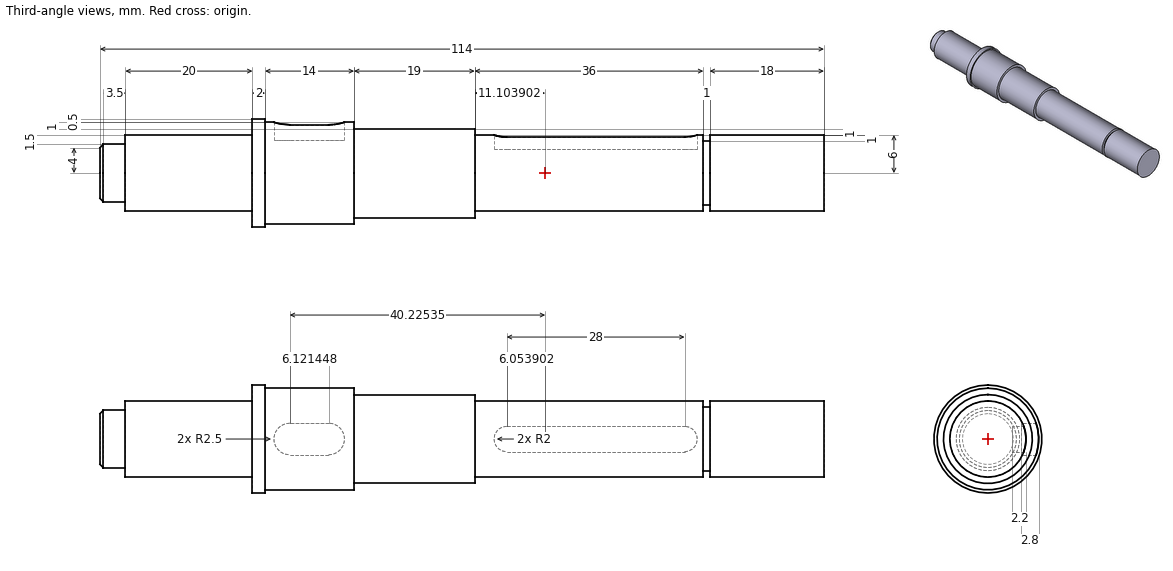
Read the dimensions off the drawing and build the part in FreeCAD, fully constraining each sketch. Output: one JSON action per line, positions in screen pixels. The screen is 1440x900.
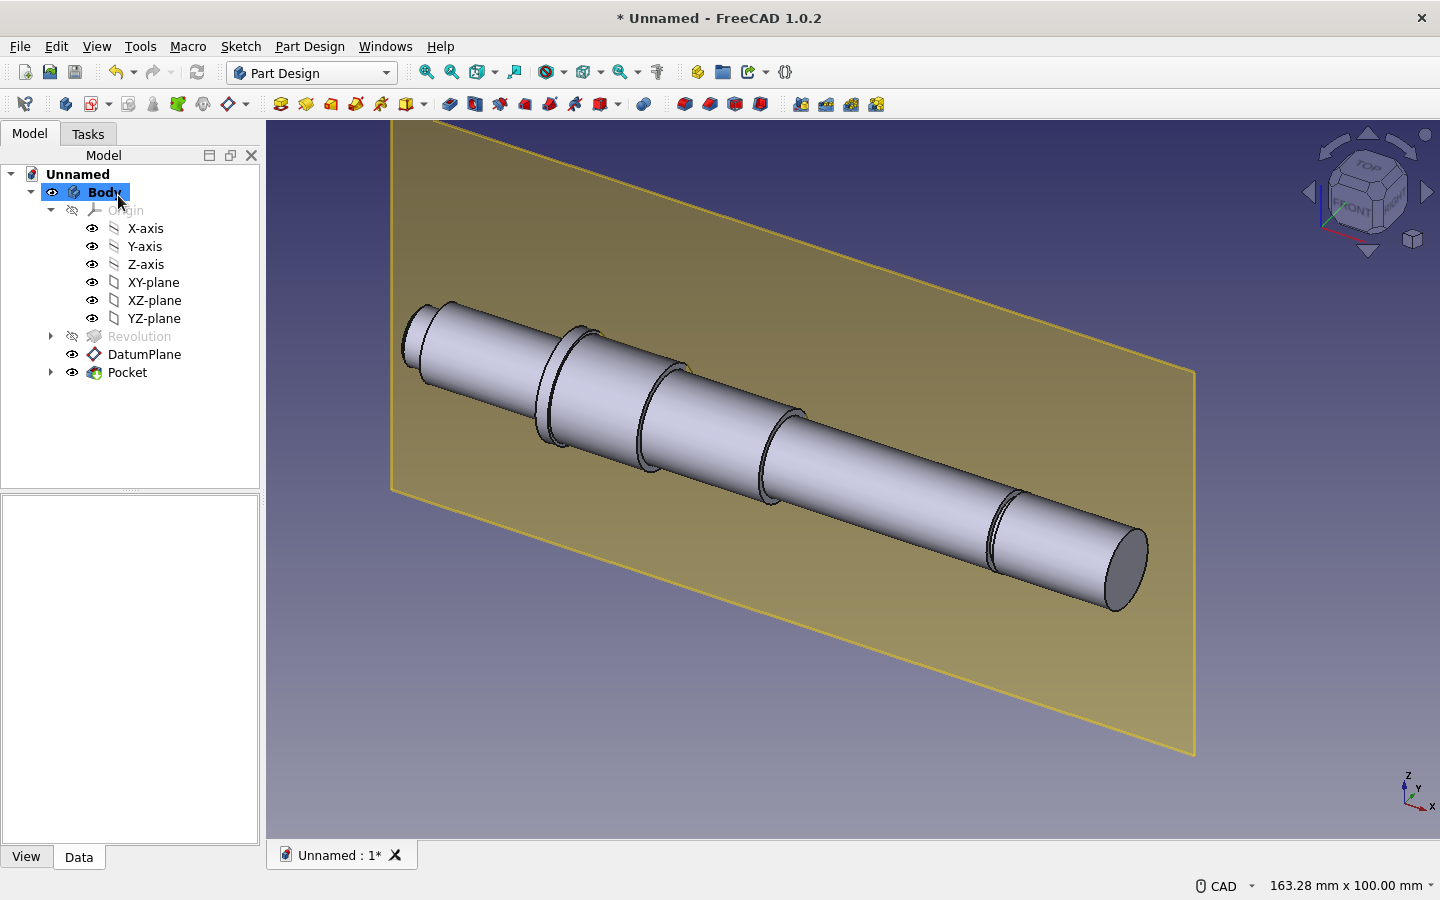
{"action": "left_click", "coordinate": [117, 354]}
{"action": "key", "text": "space"}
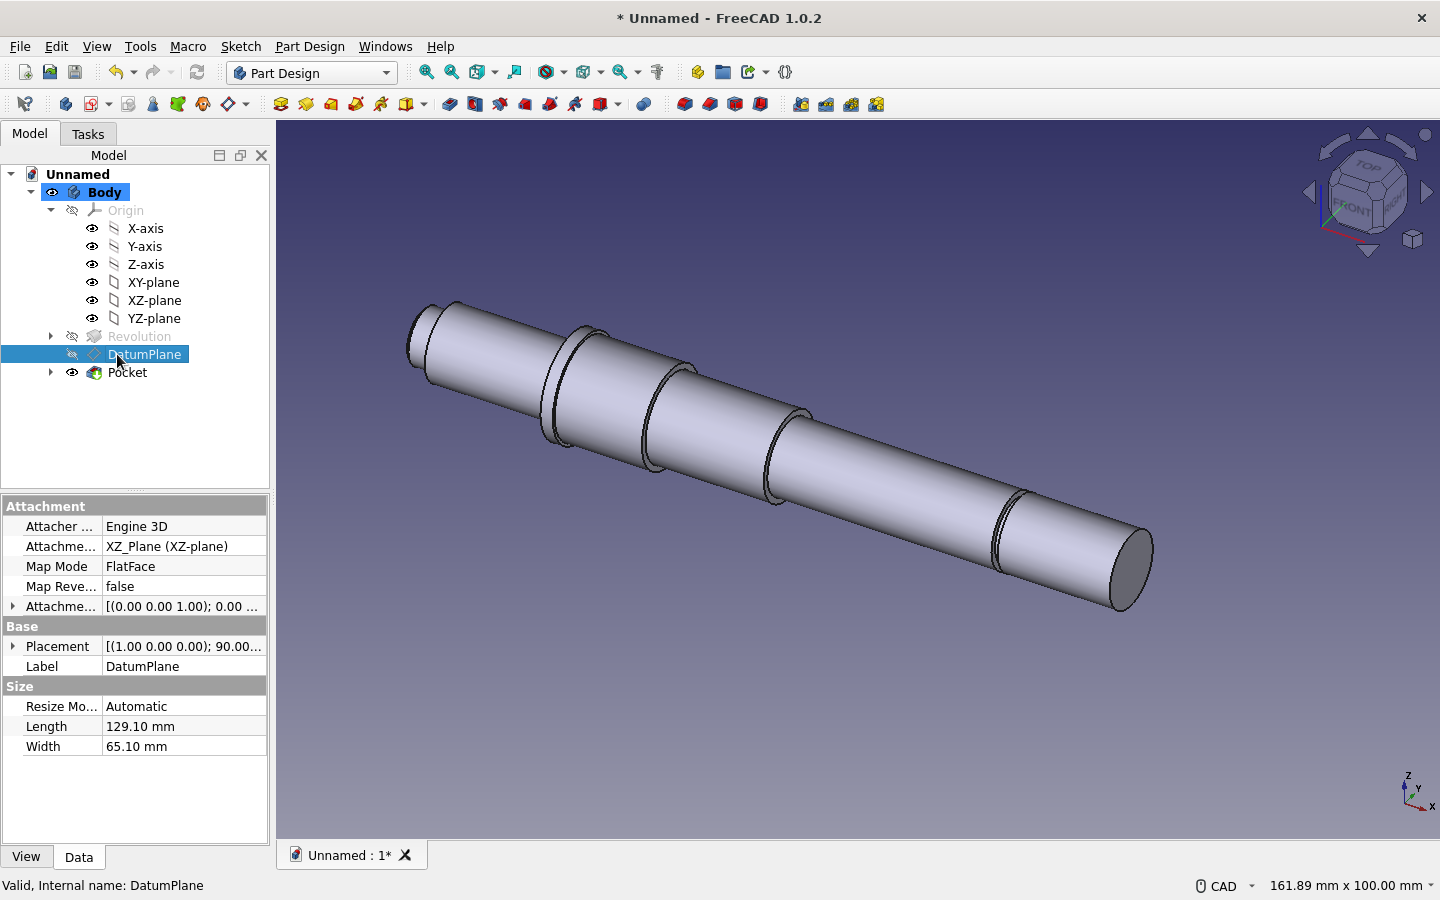
{"action": "left_click", "coordinate": [137, 300]}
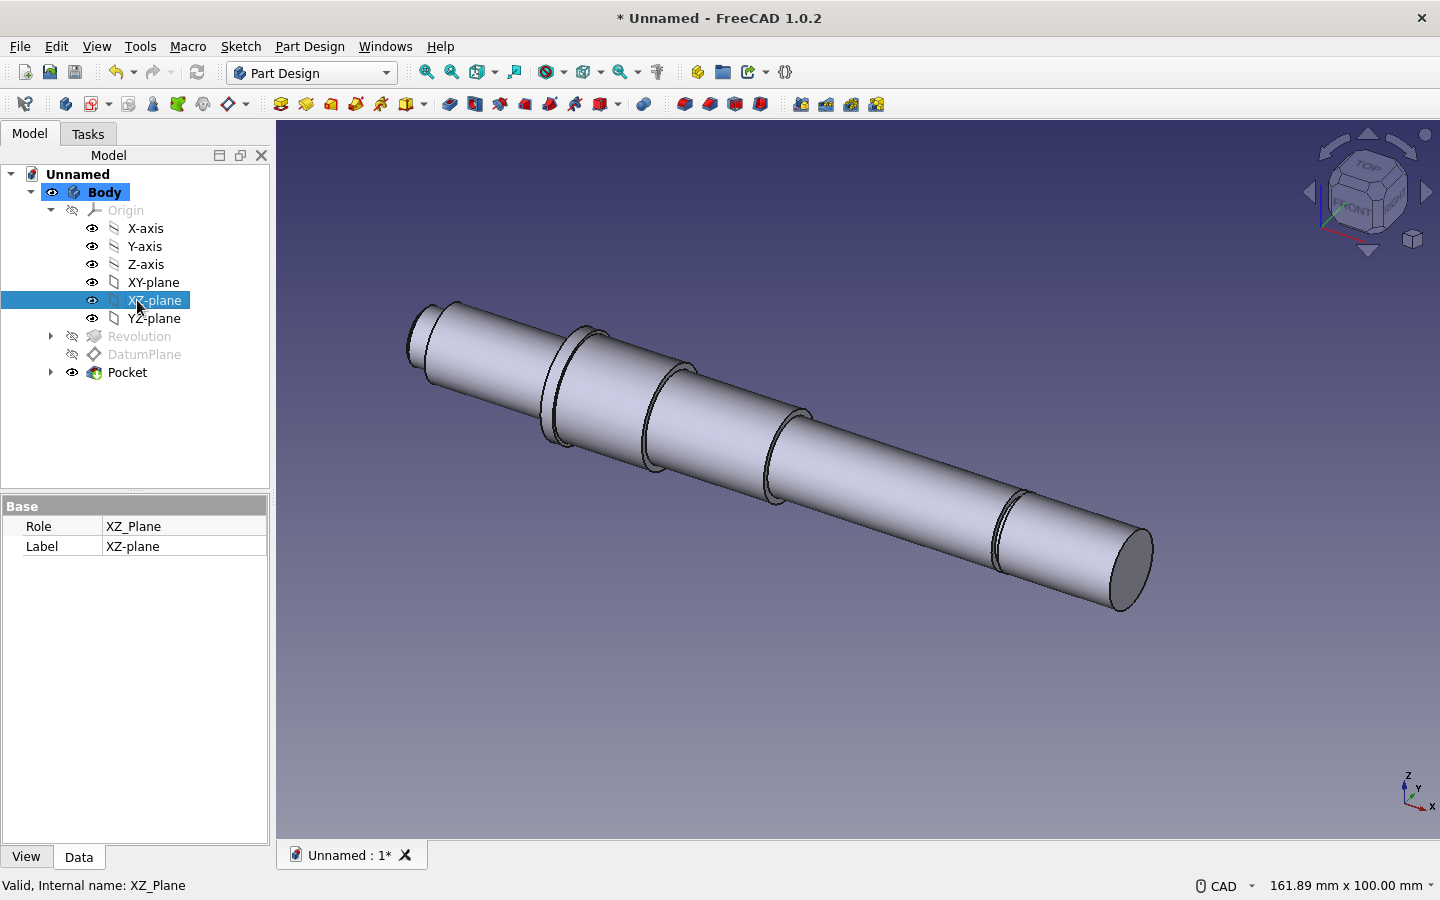
{"action": "left_click", "coordinate": [228, 104]}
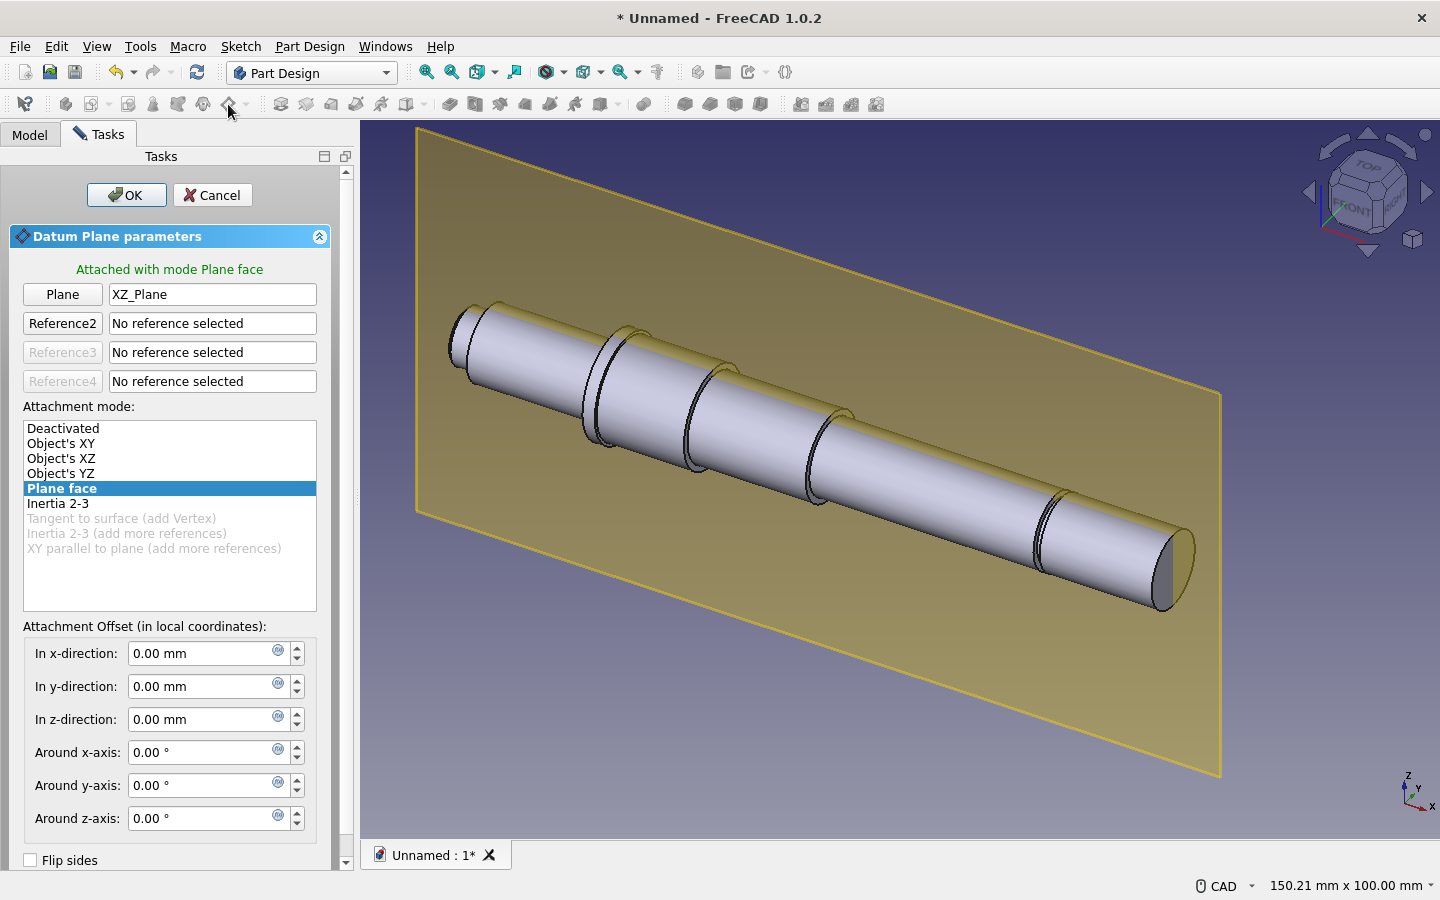
{"action": "triple_click", "coordinate": [210, 720]}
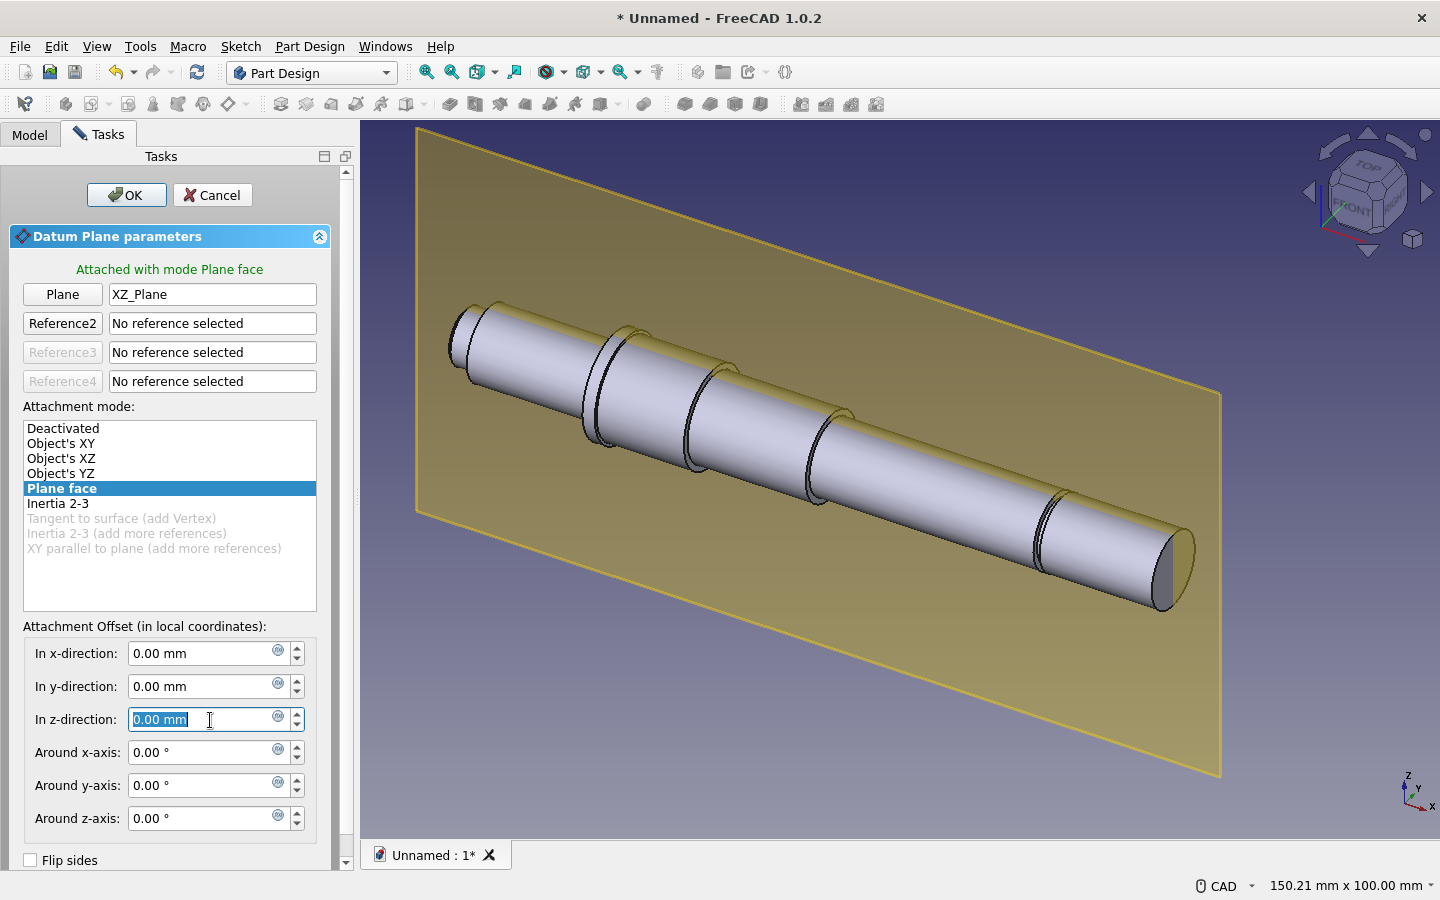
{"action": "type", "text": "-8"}
{"action": "key", "text": "Tab"}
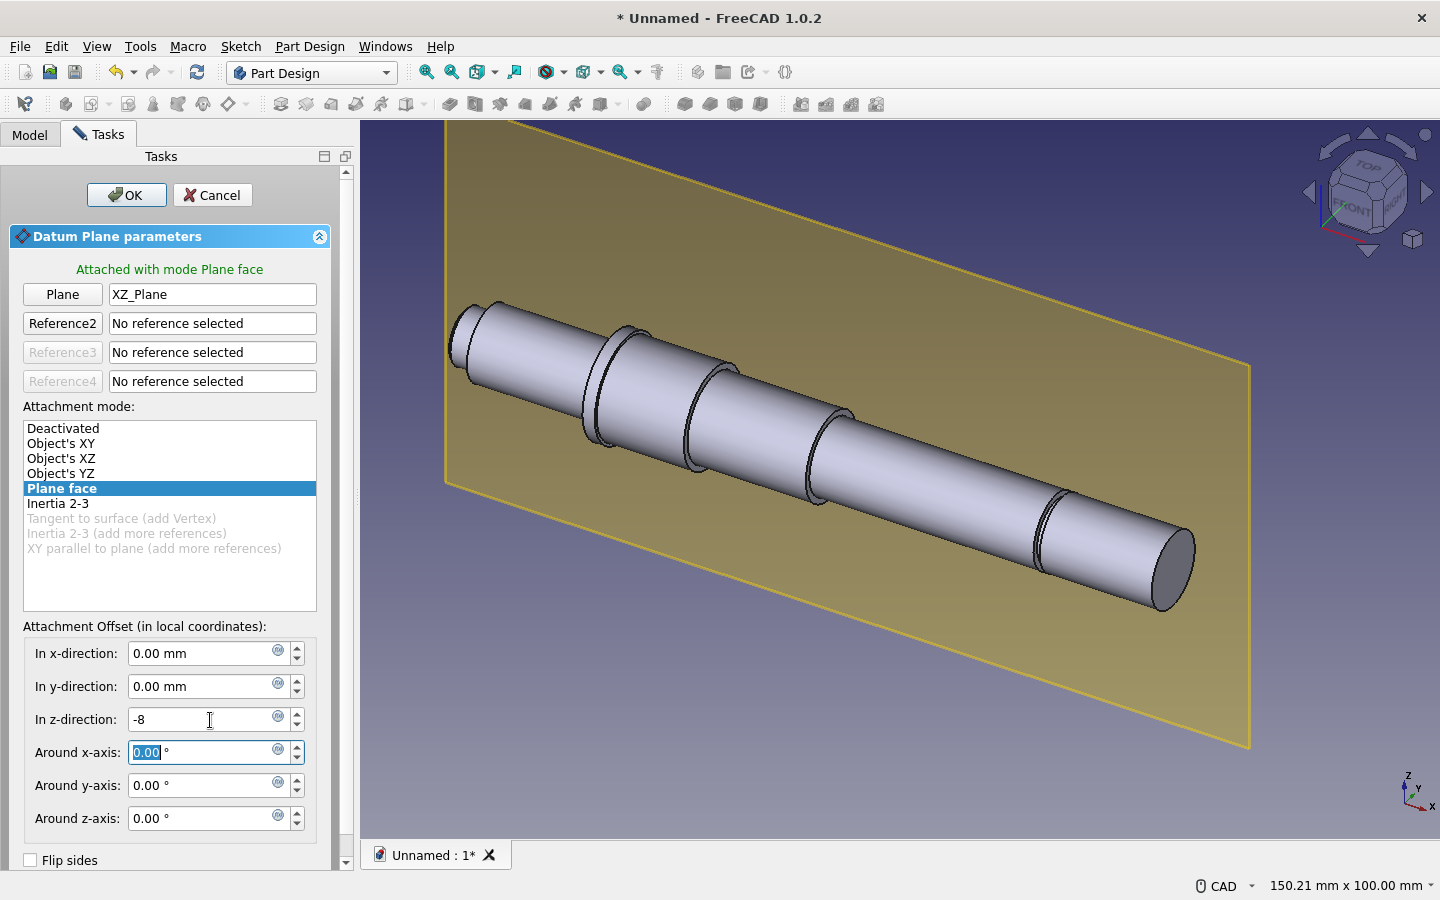
{"action": "left_click", "coordinate": [127, 195]}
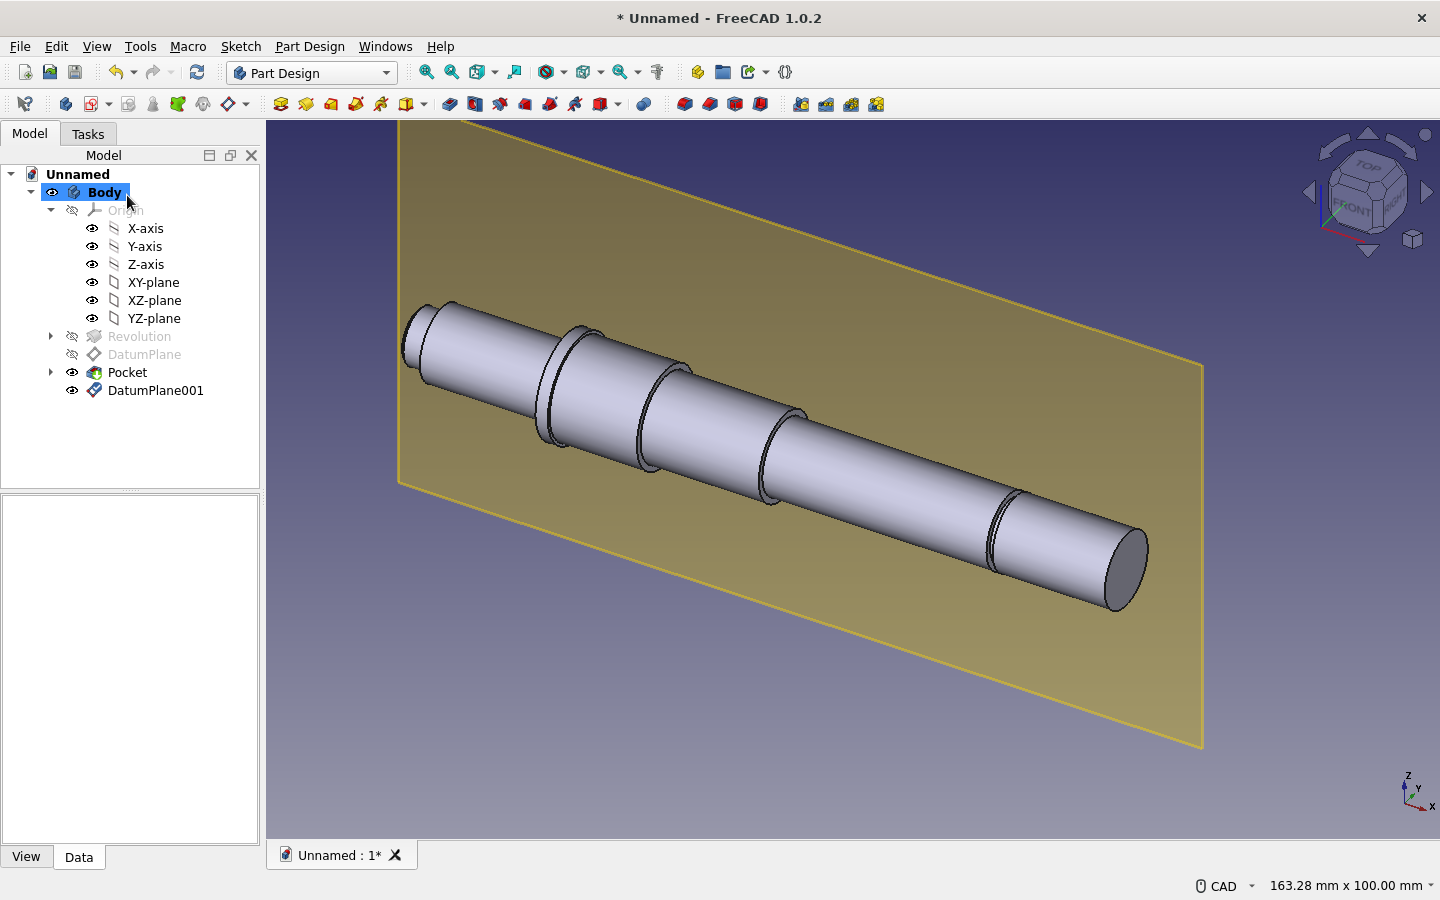
{"action": "left_click", "coordinate": [117, 390]}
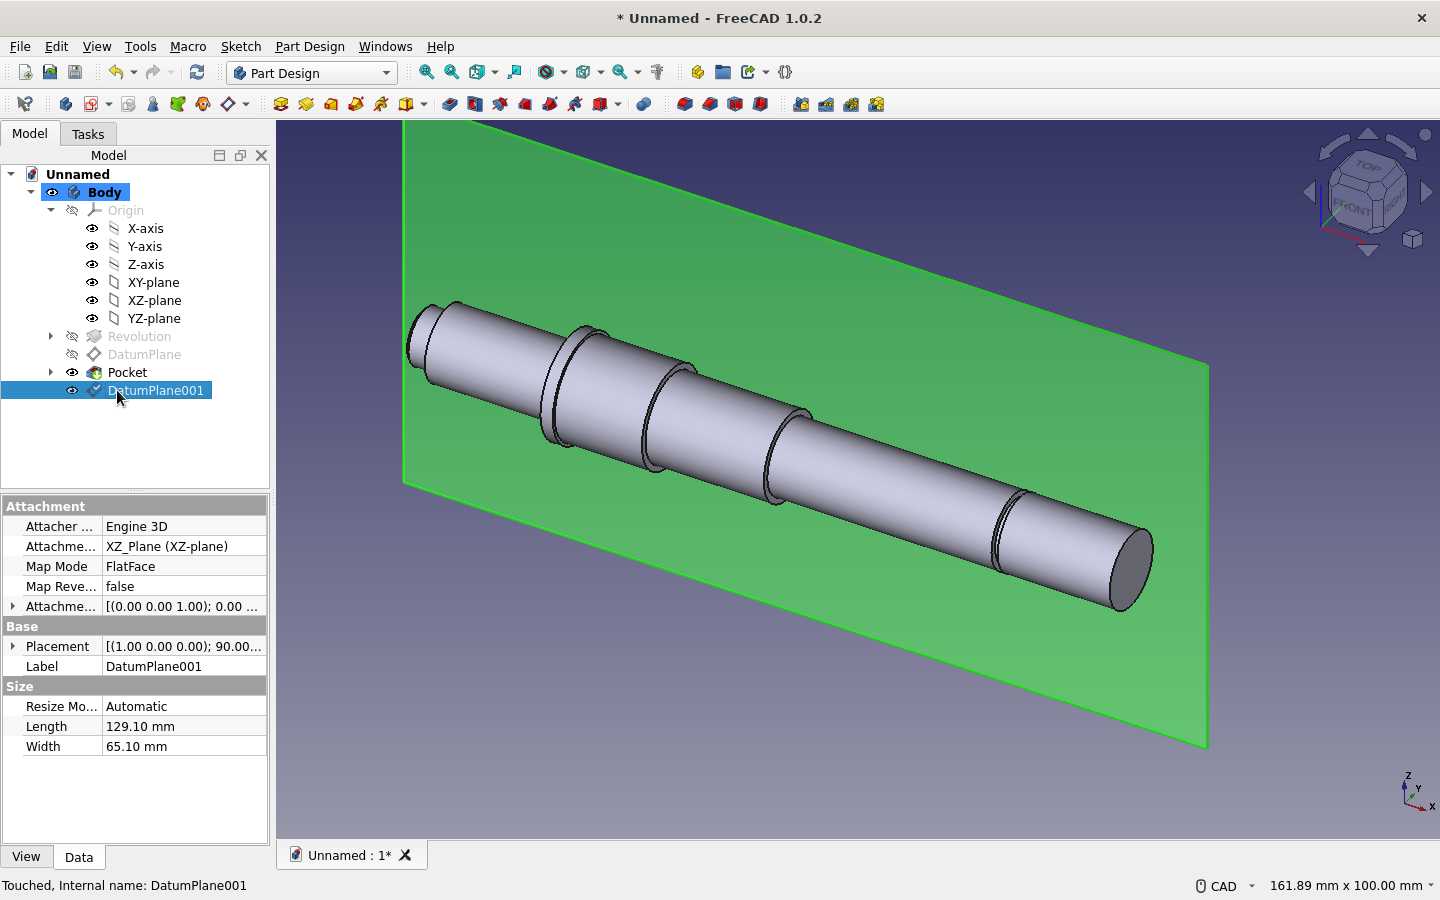
{"action": "left_click", "coordinate": [90, 104]}